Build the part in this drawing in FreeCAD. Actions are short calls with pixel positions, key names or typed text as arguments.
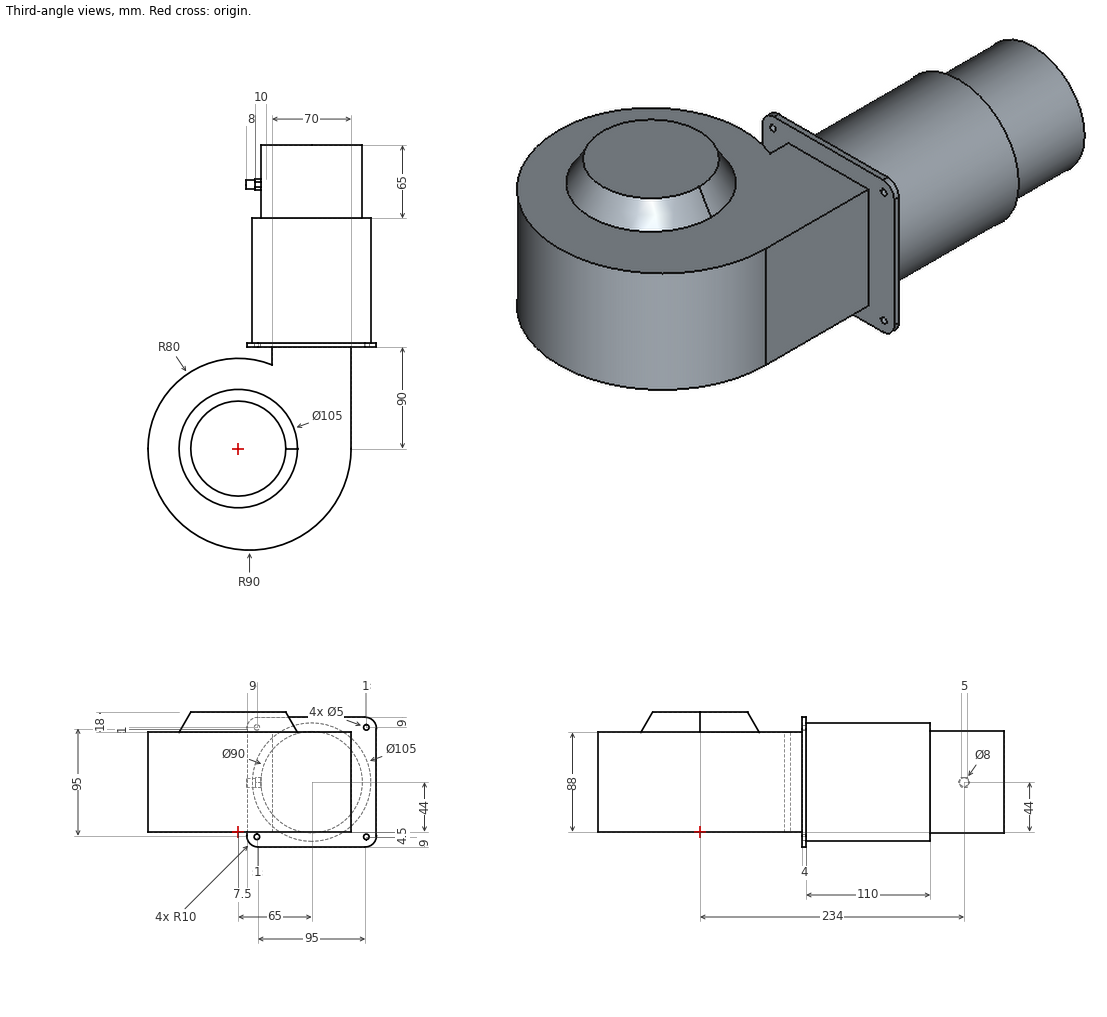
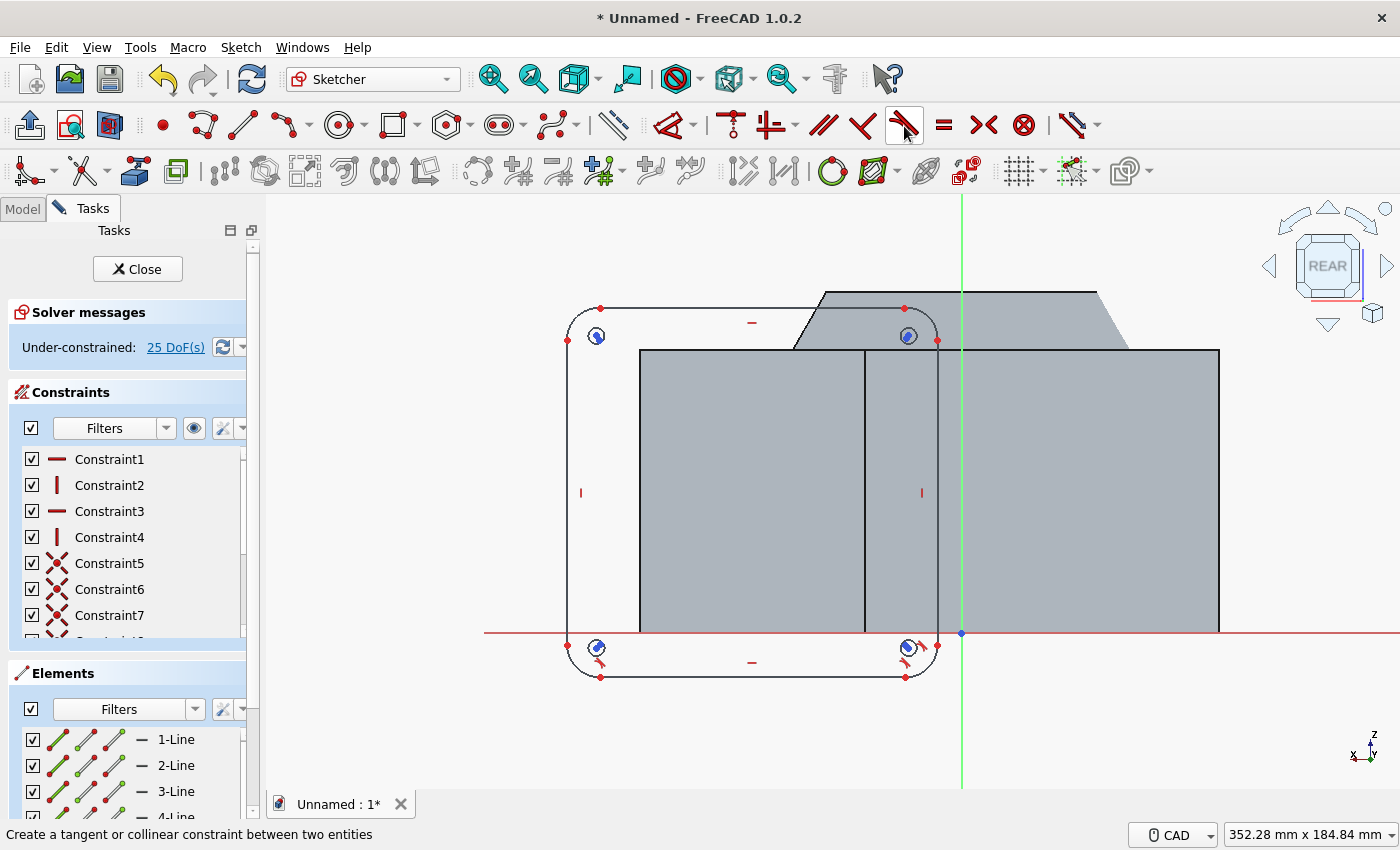
click(938, 554)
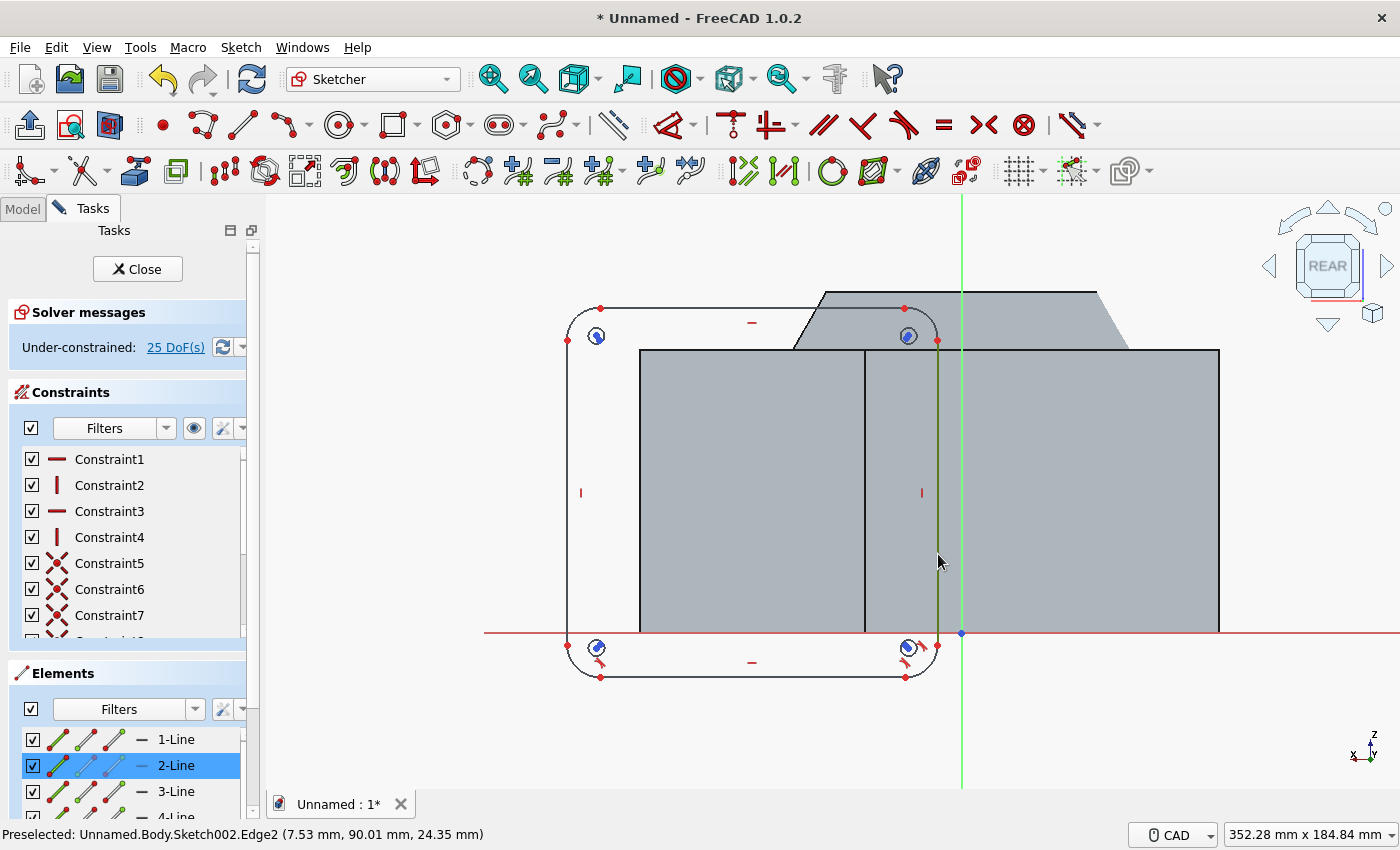
click(934, 325)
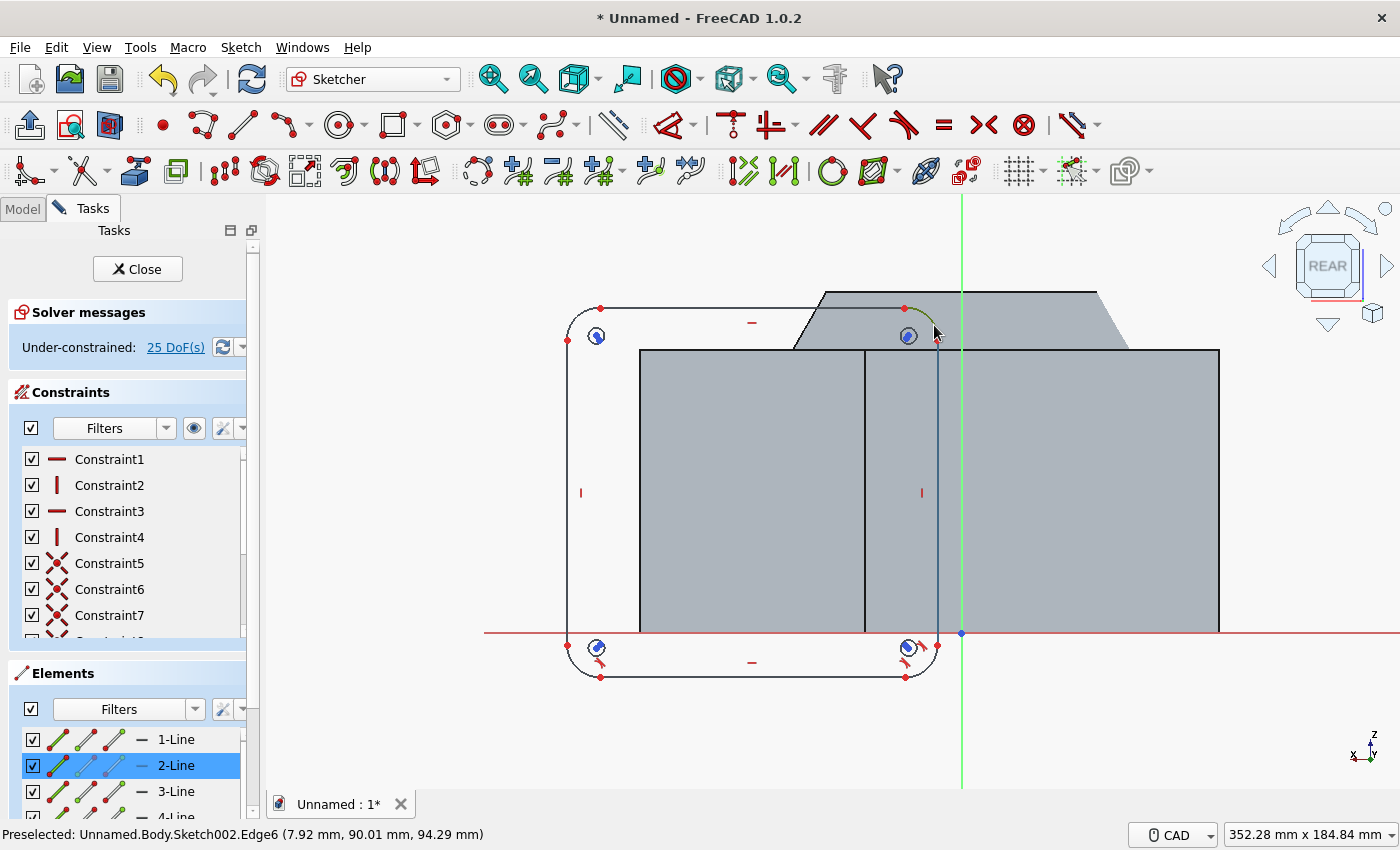
click(904, 126)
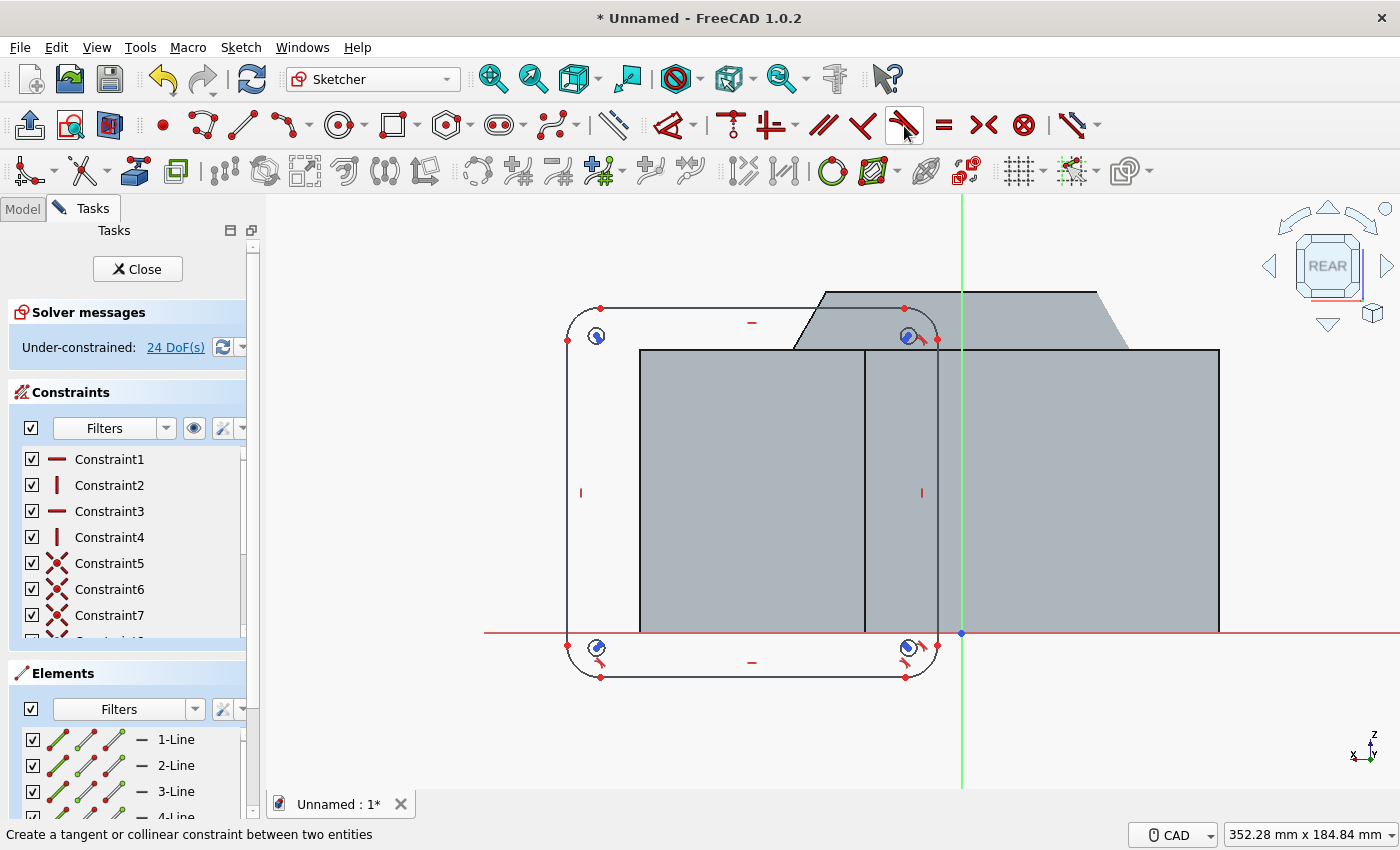
click(813, 308)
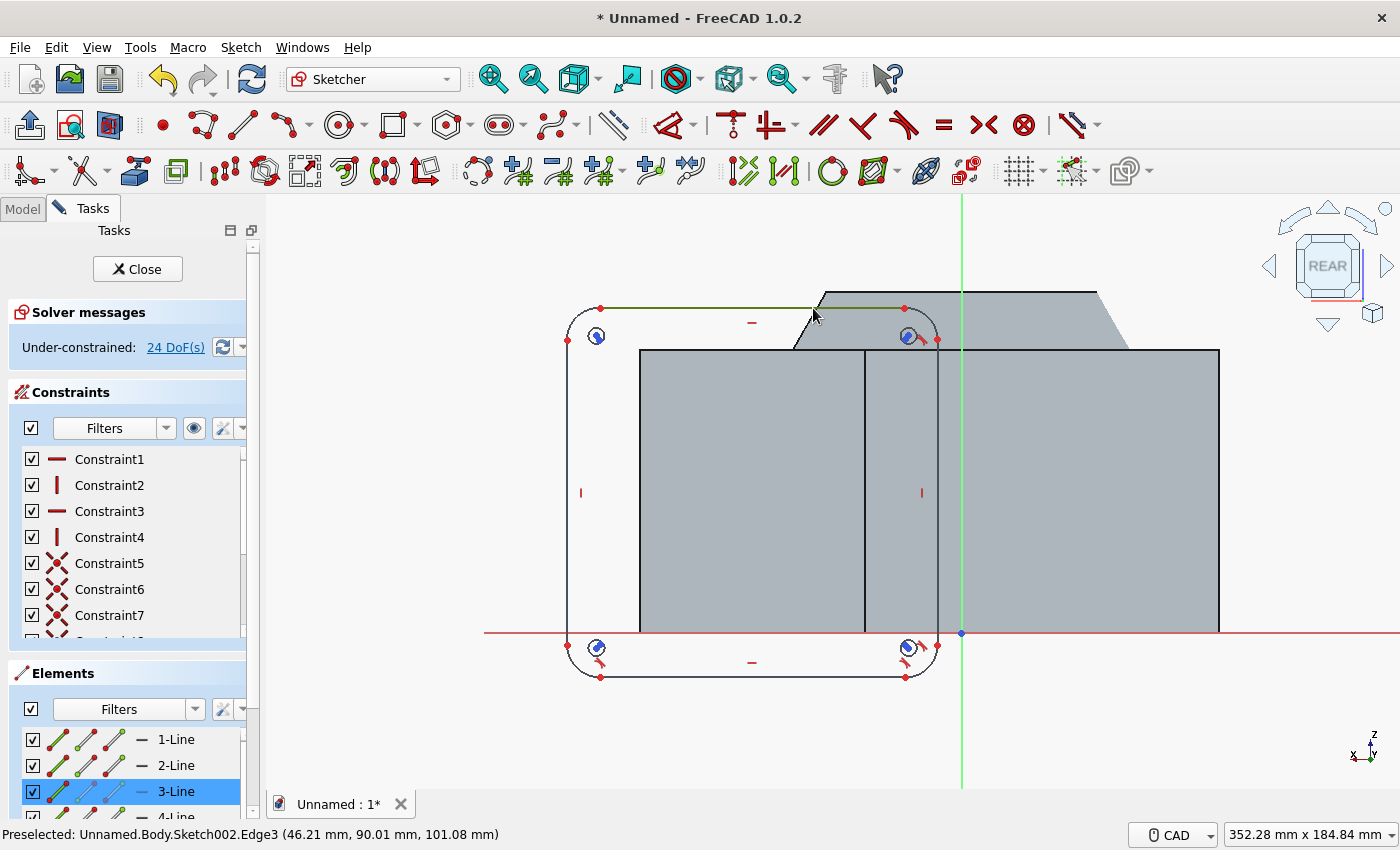
click(934, 325)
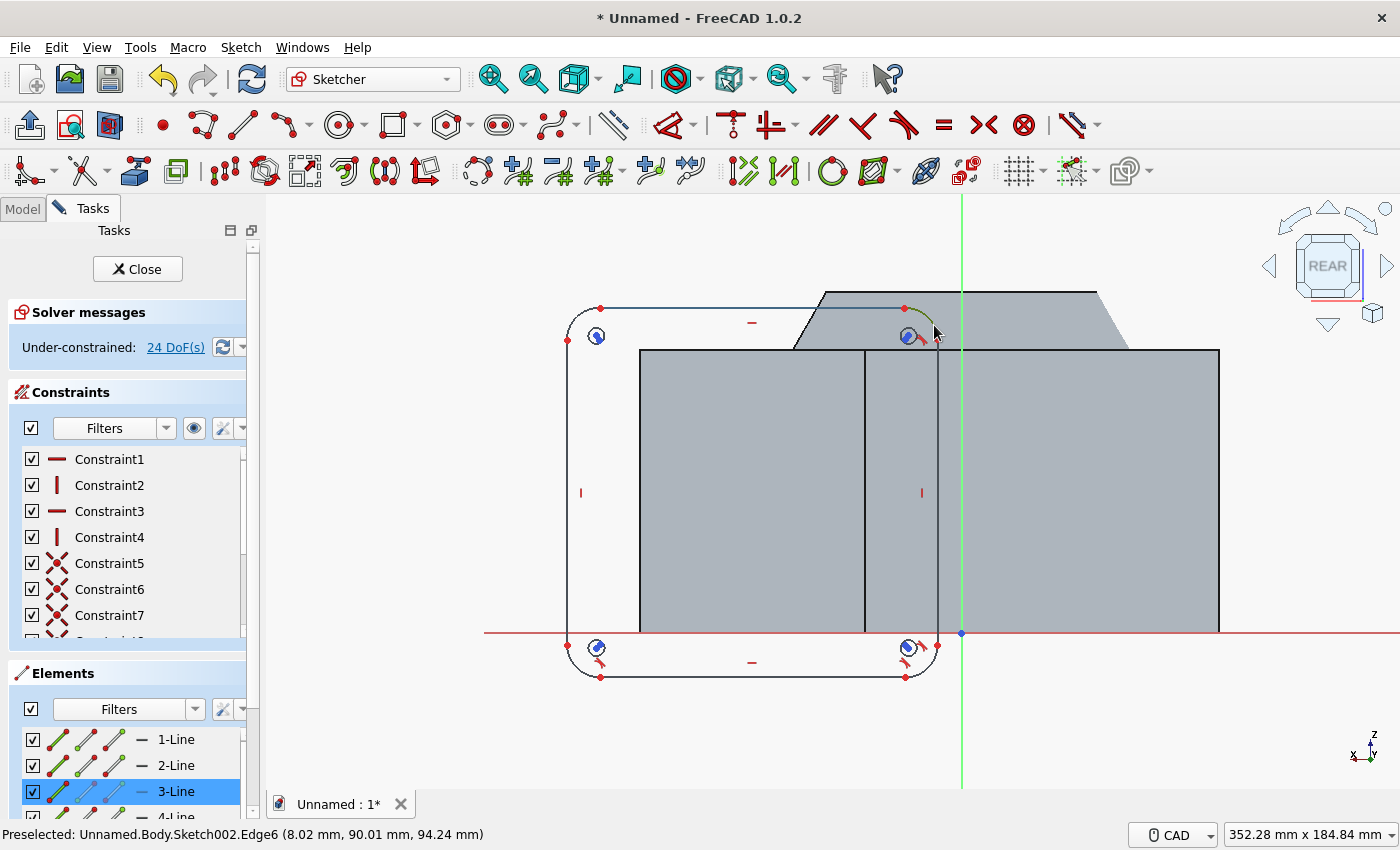
click(904, 126)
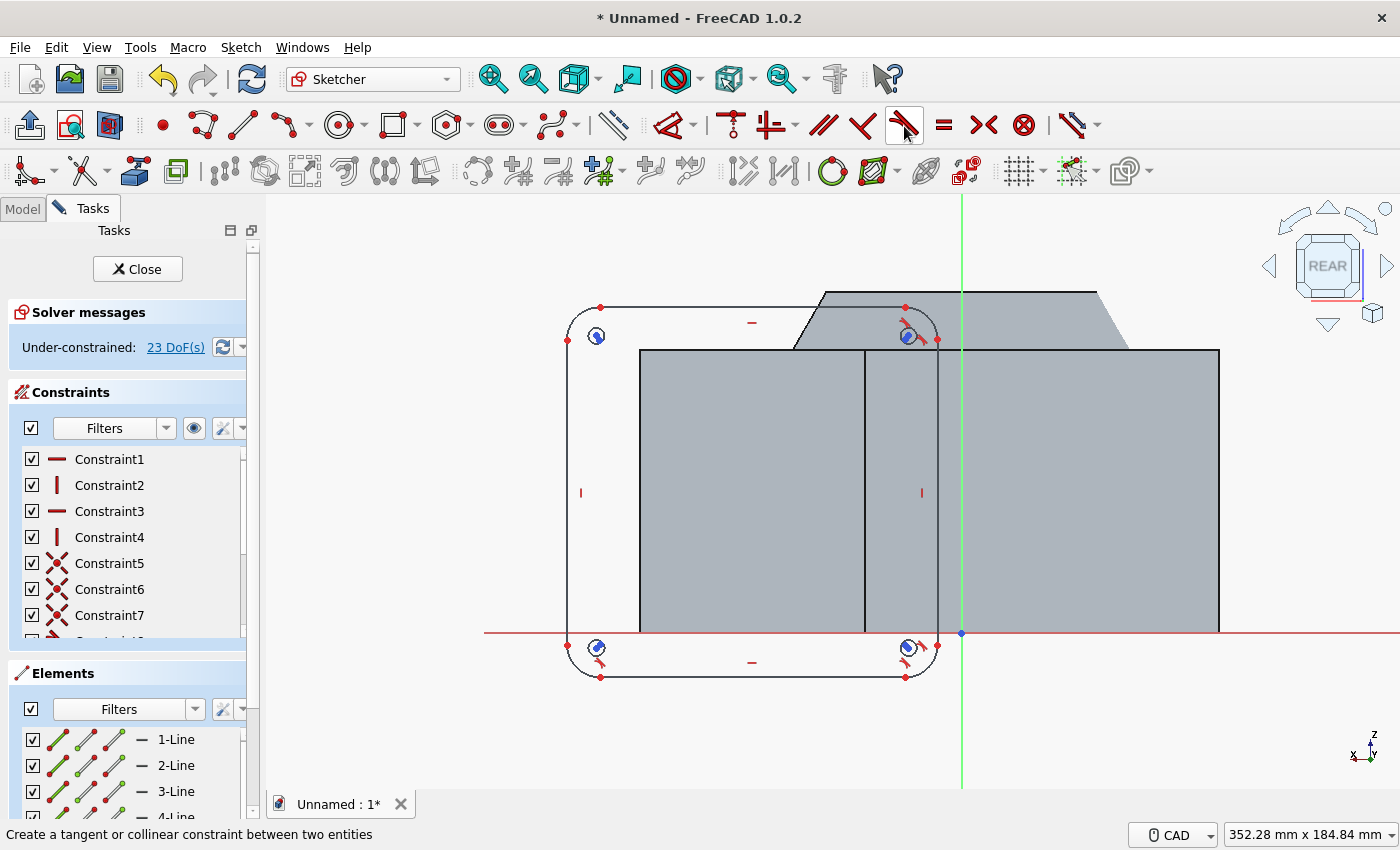
click(814, 307)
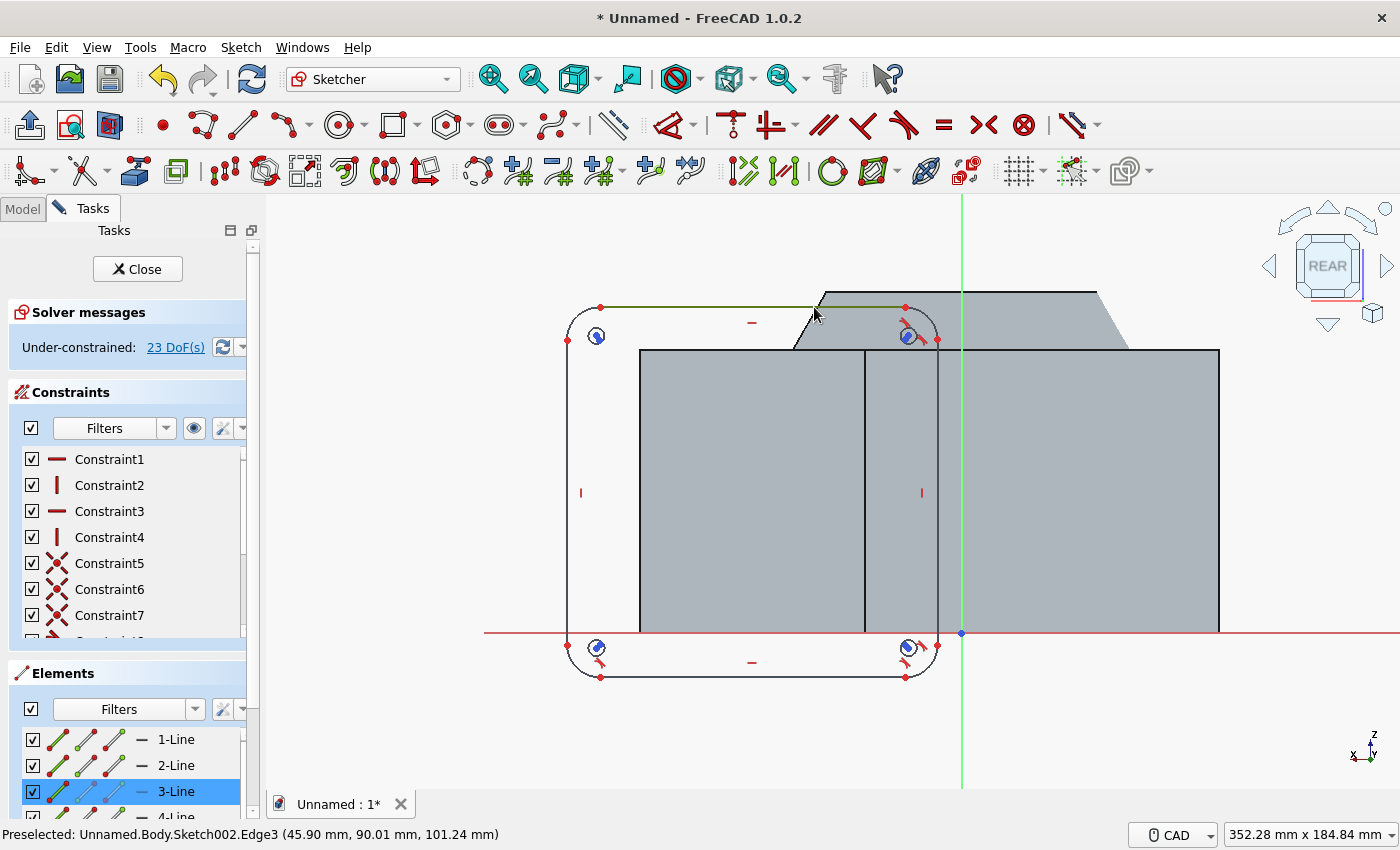
click(585, 311)